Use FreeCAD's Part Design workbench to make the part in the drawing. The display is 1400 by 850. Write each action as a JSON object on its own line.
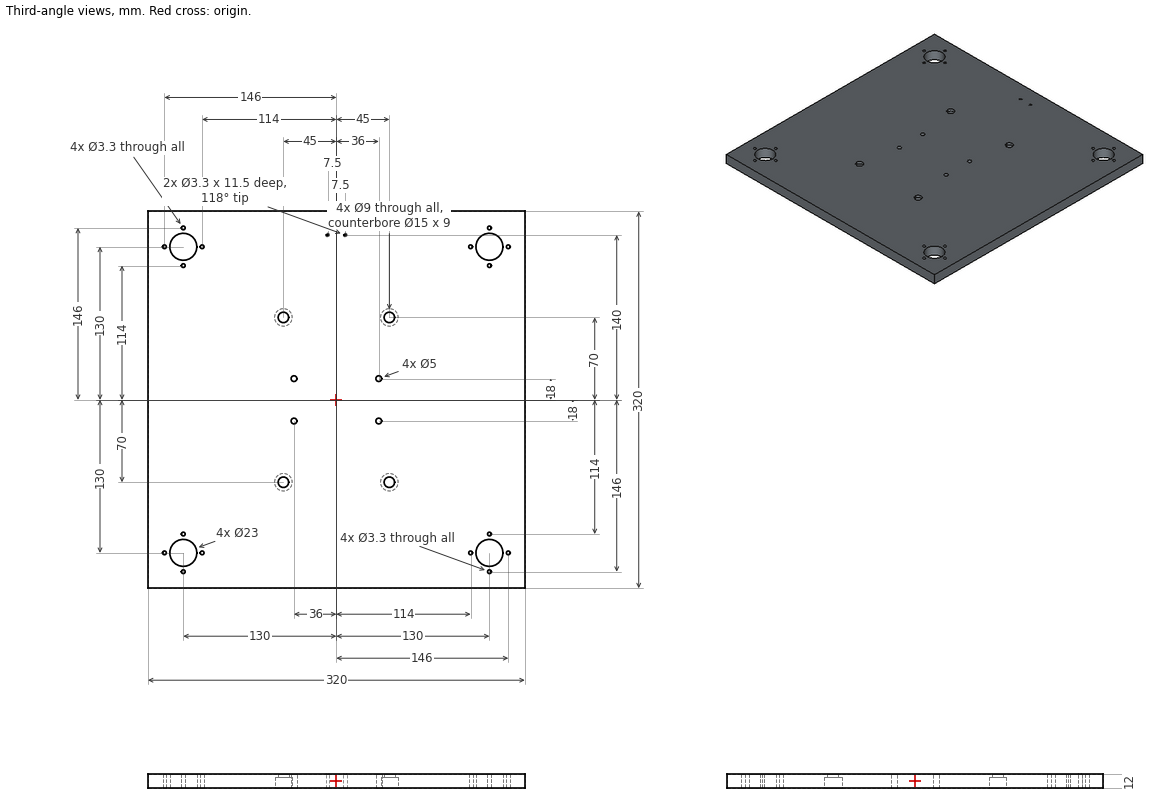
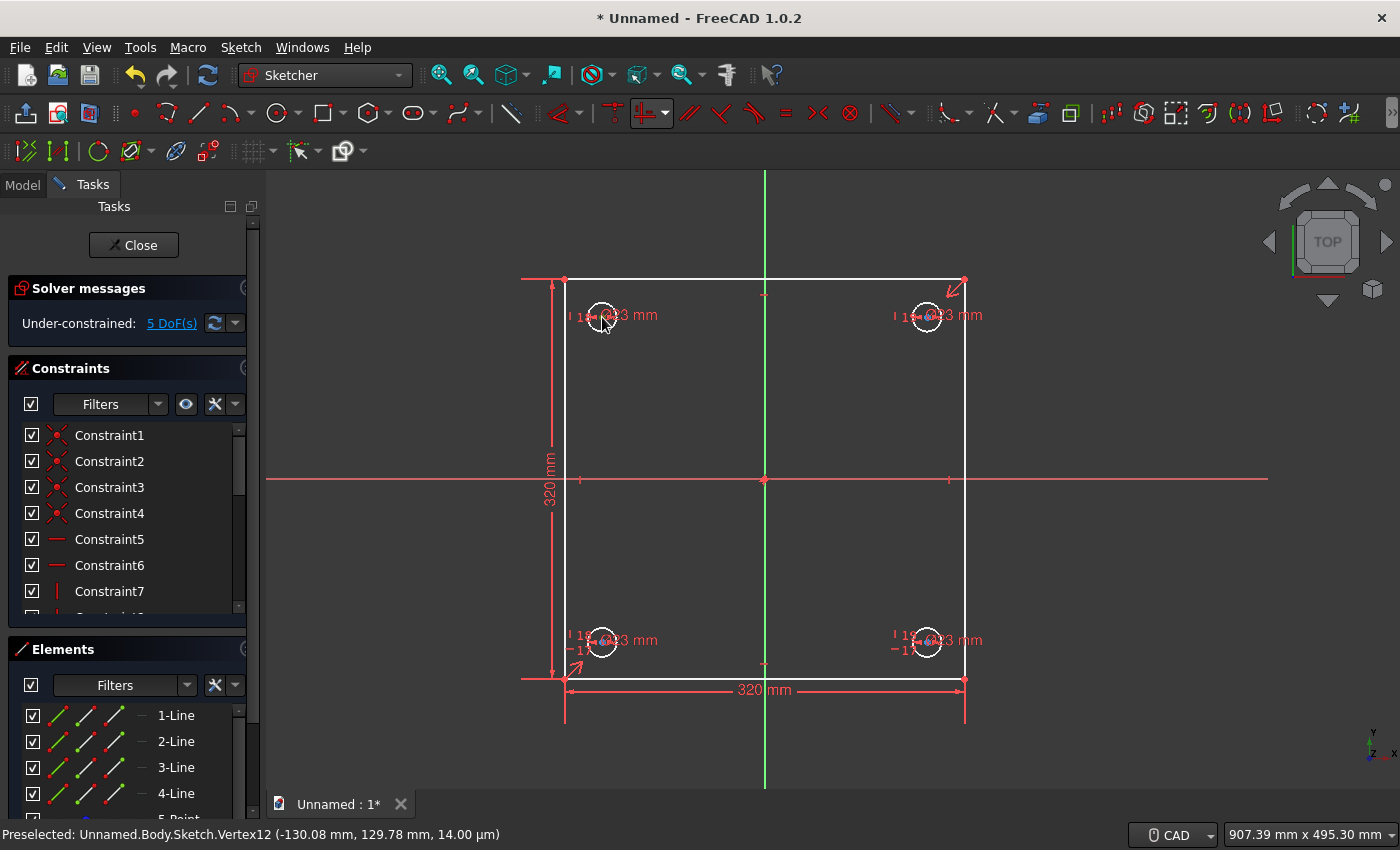
{"action": "left_click", "coordinate": [927, 317]}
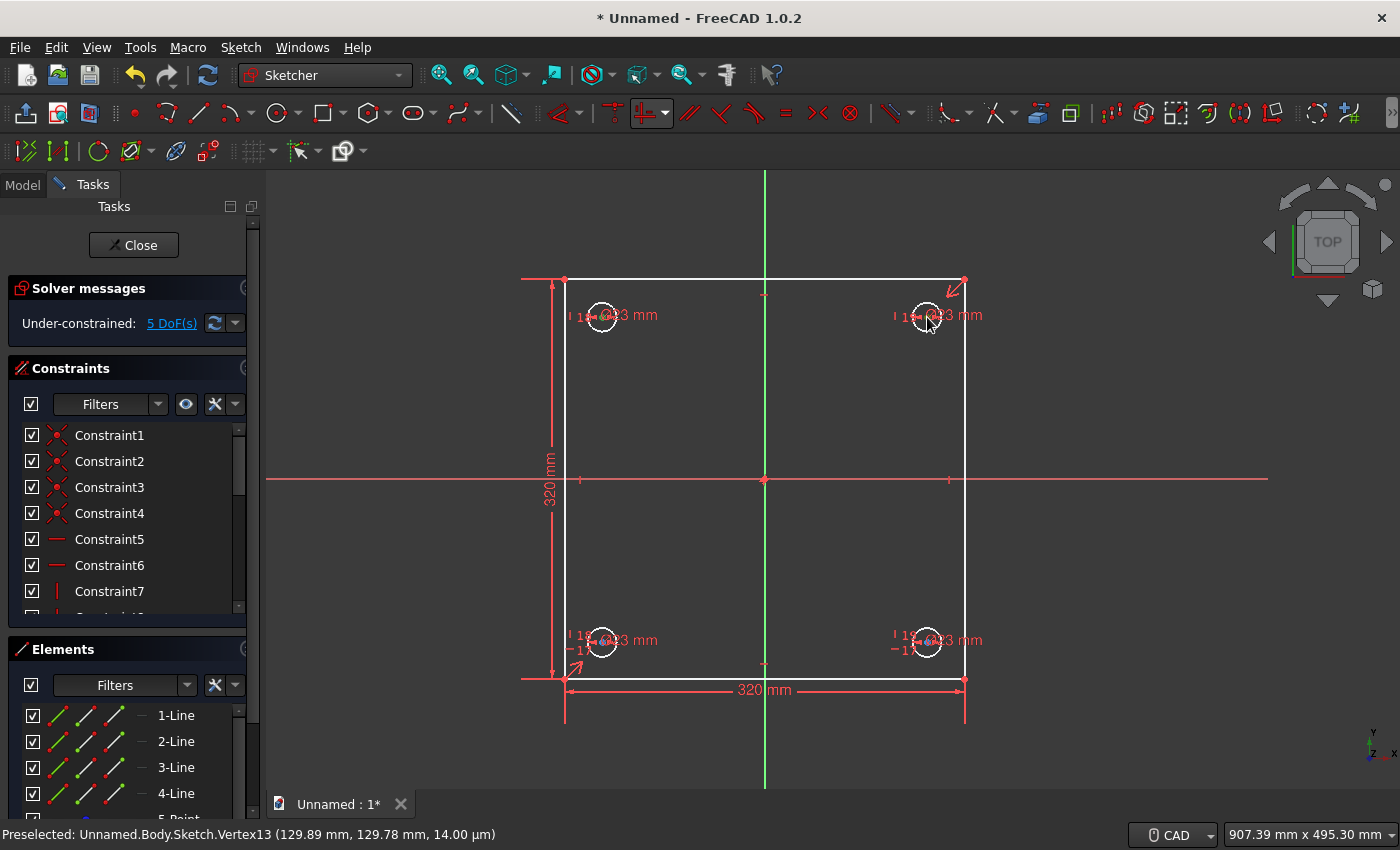
{"action": "left_click", "coordinate": [668, 114]}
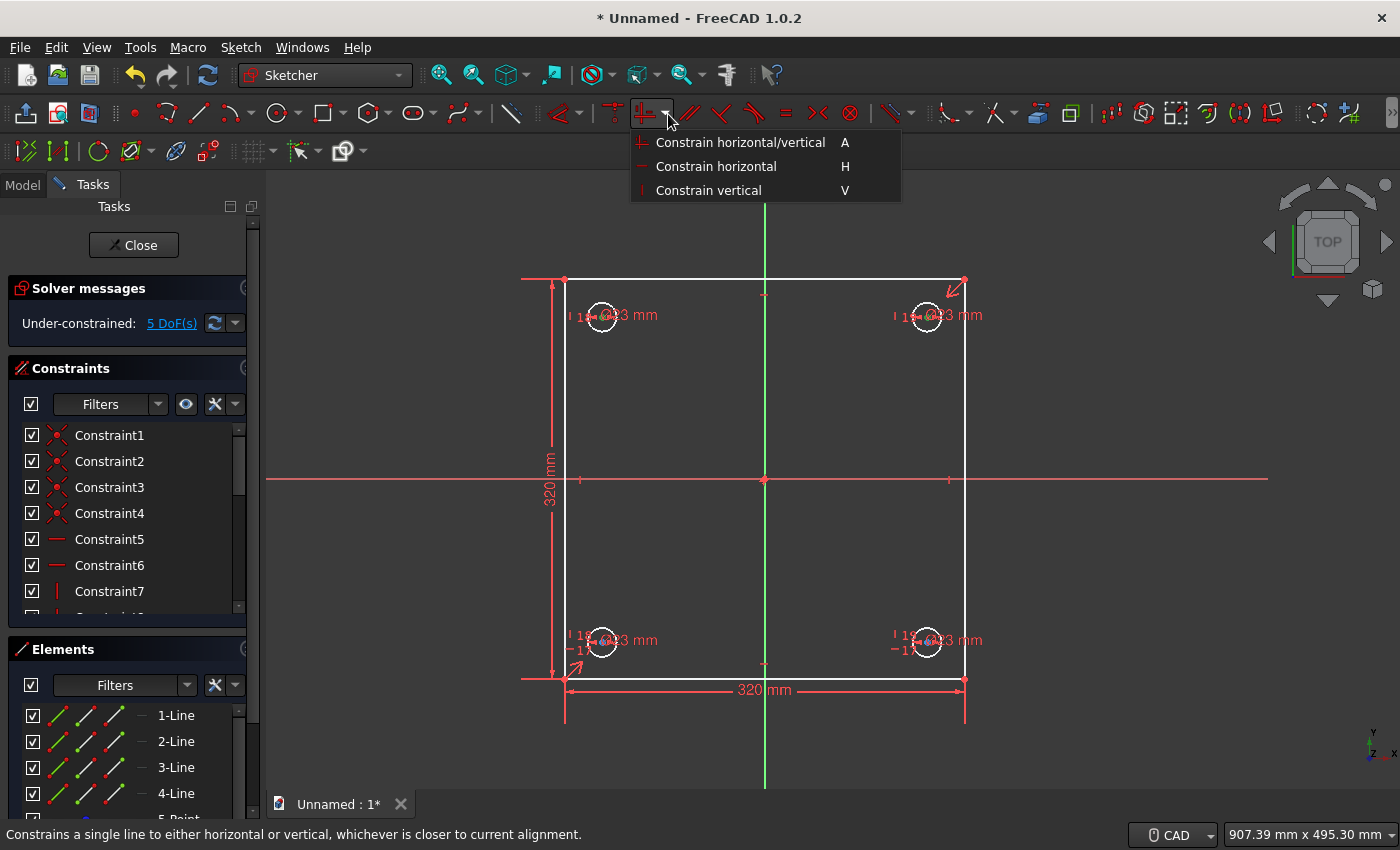
{"action": "left_click", "coordinate": [766, 166]}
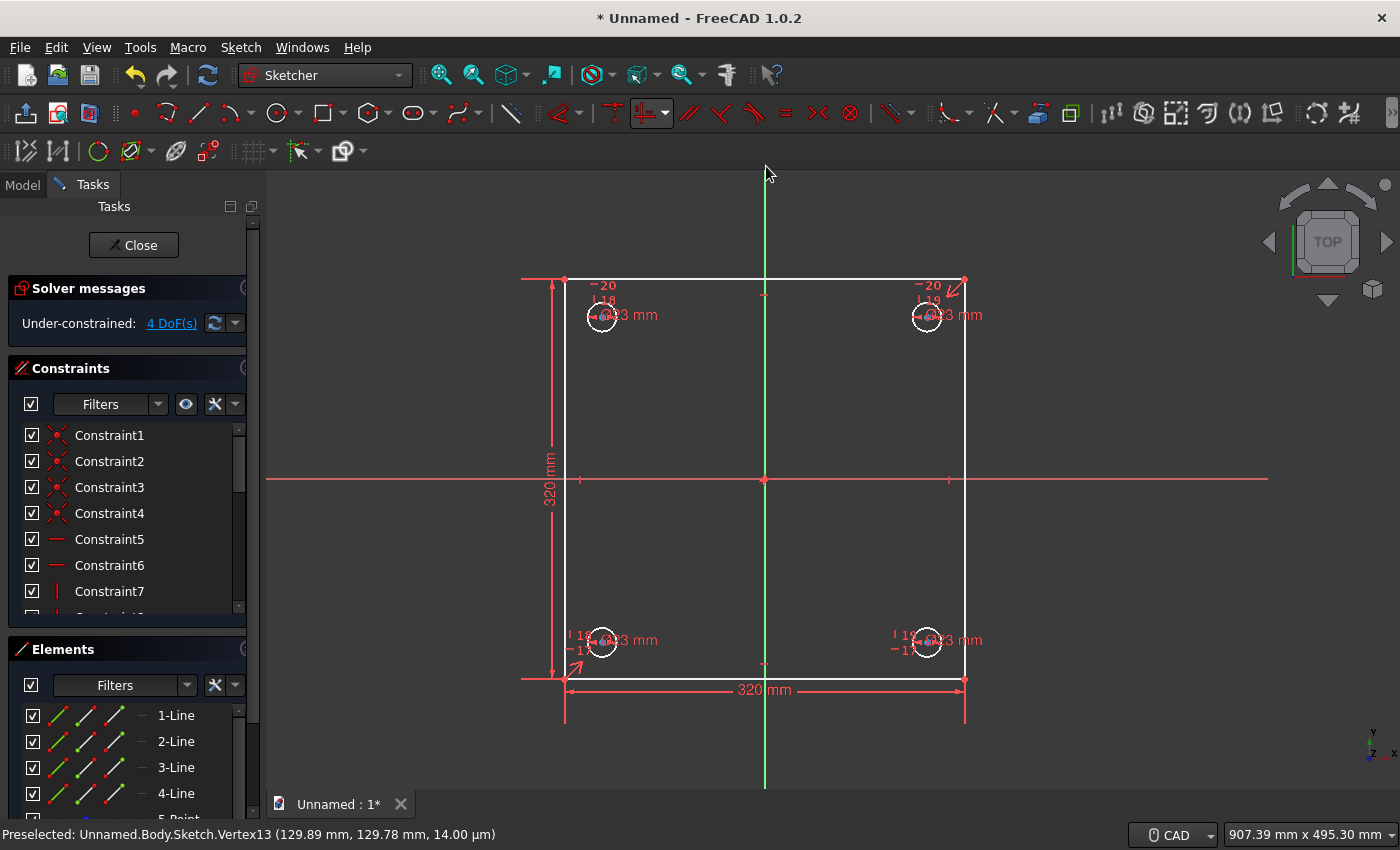
{"action": "left_click", "coordinate": [602, 642]}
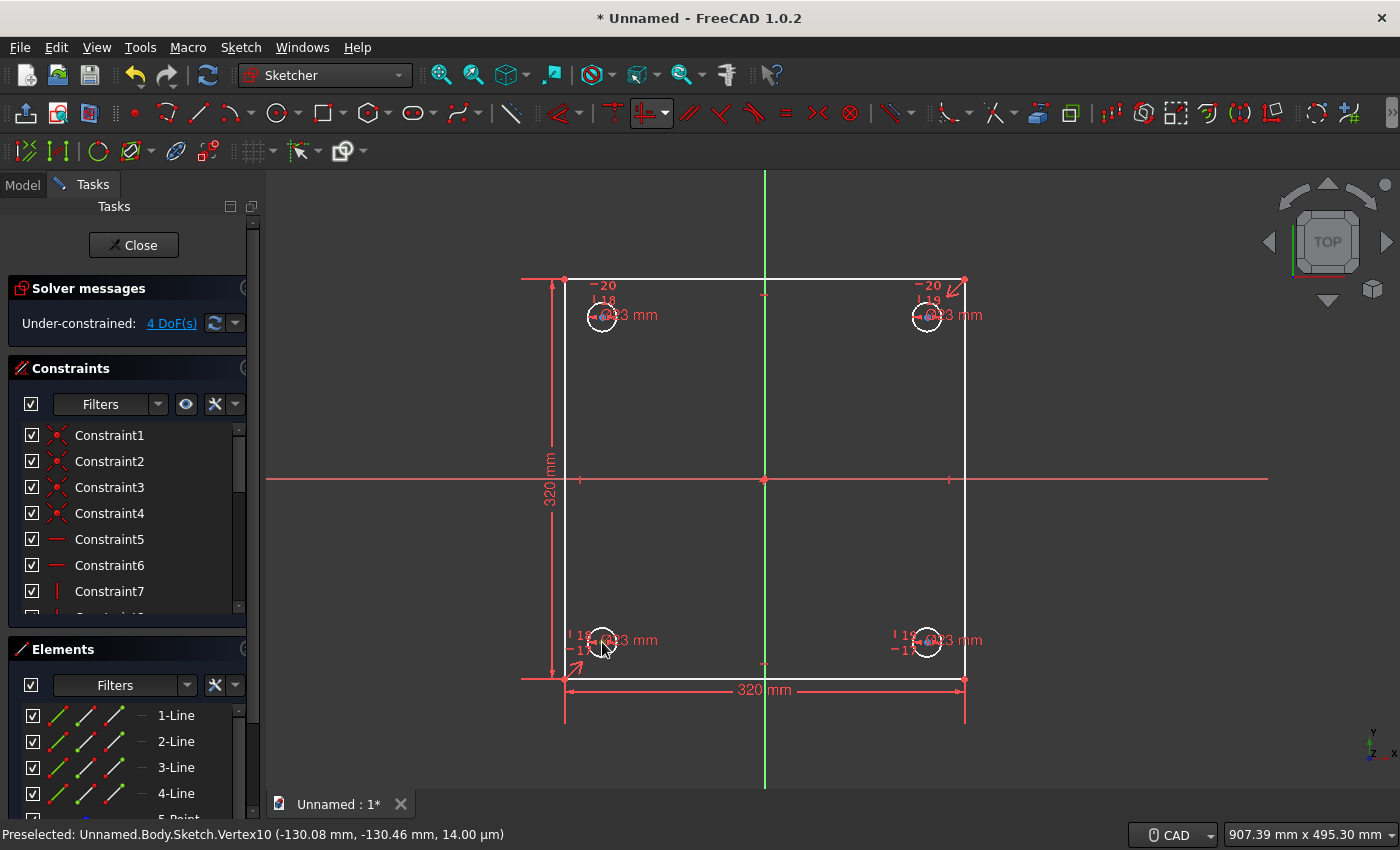
{"action": "key", "text": "l"}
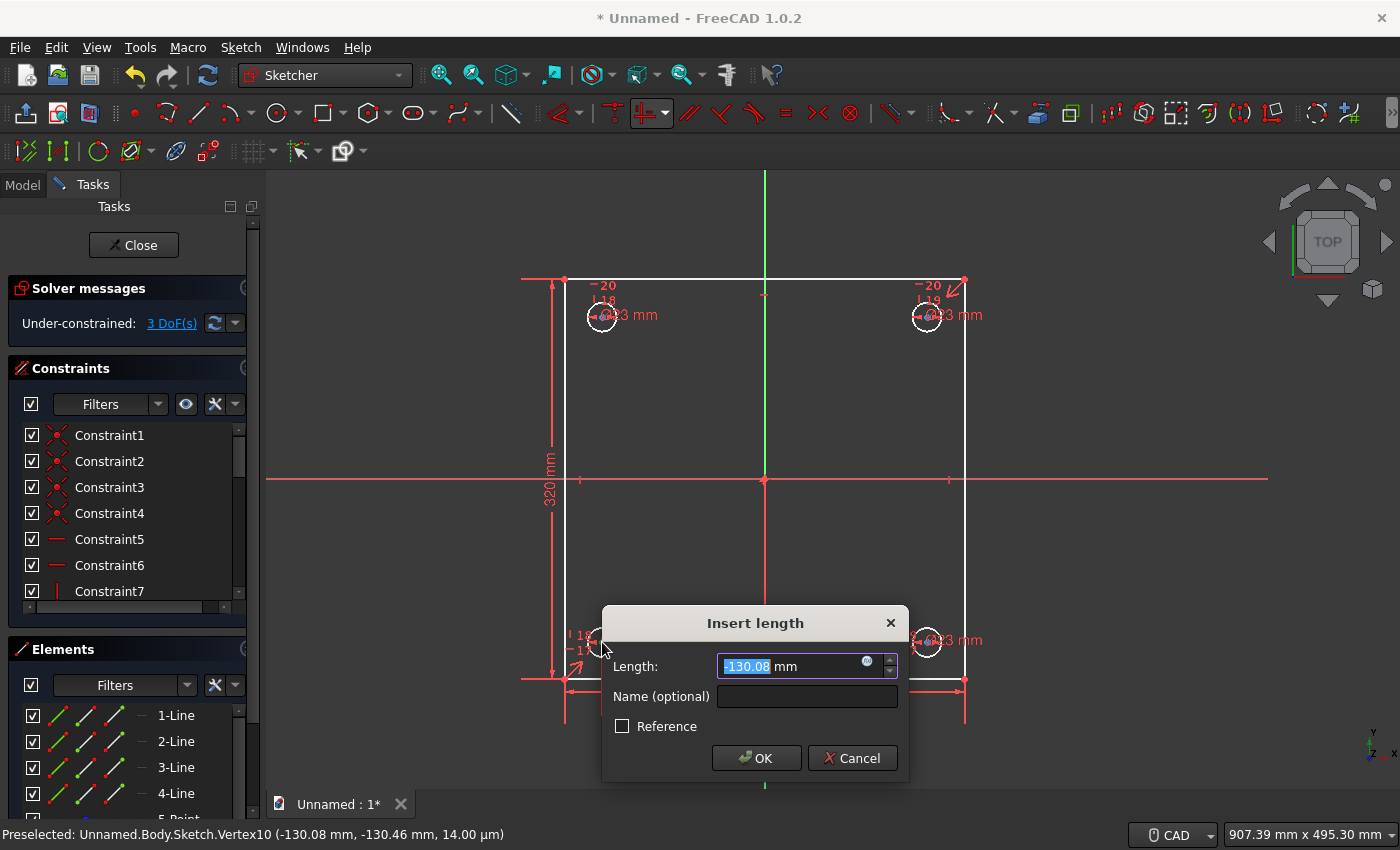
{"action": "type", "text": "-130"}
{"action": "key", "text": "Return"}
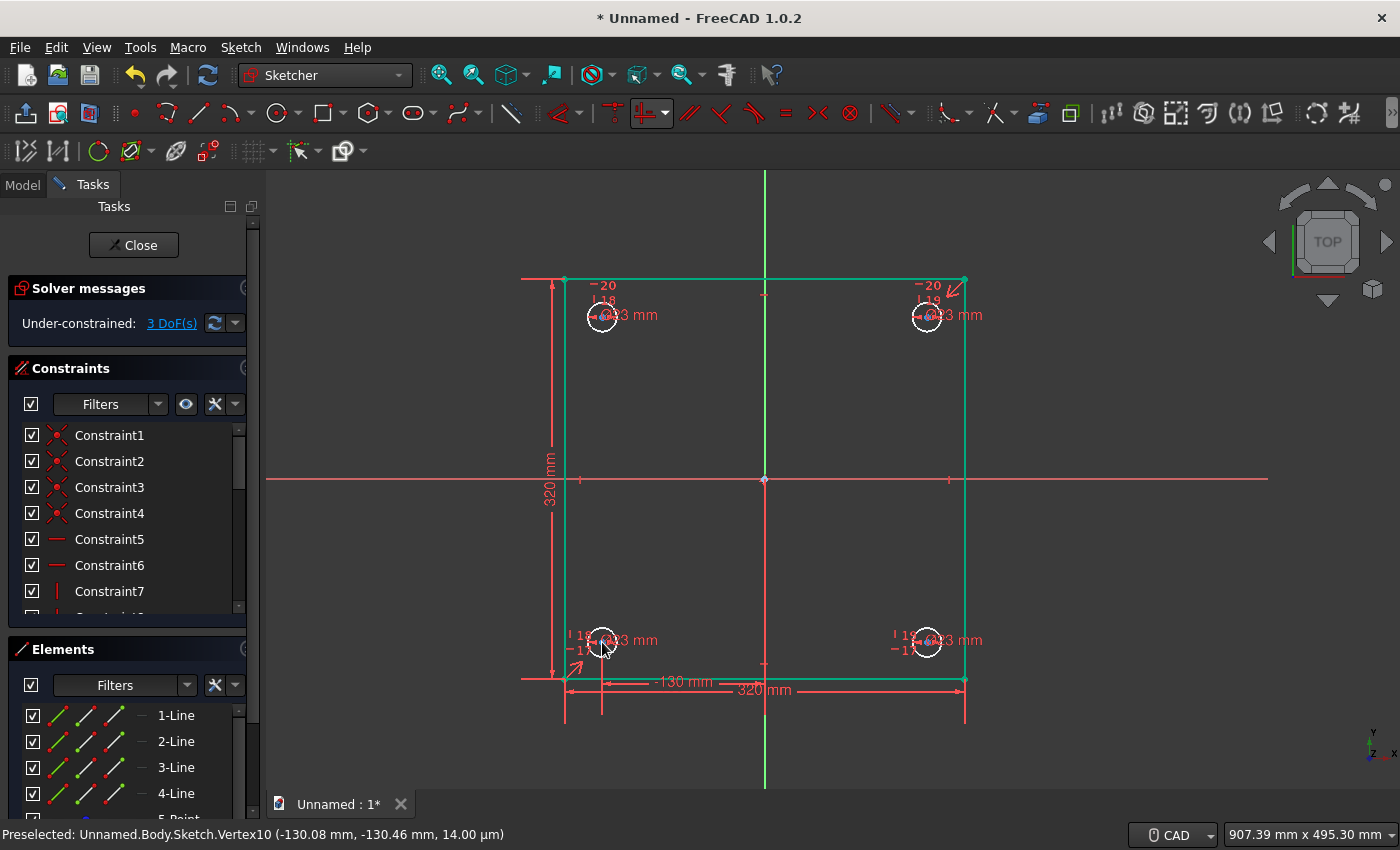
{"action": "left_click", "coordinate": [602, 642]}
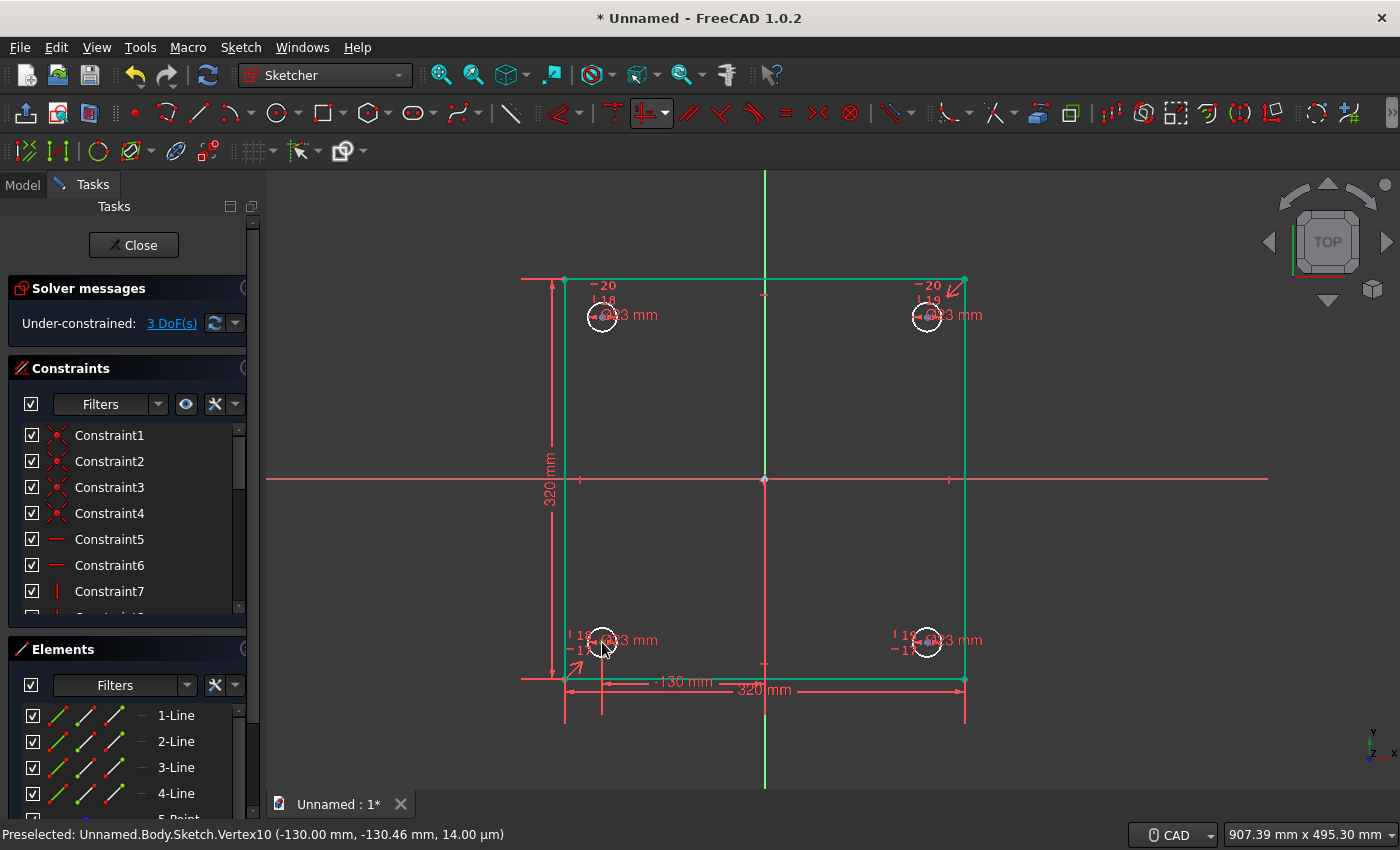
{"action": "key", "text": "i"}